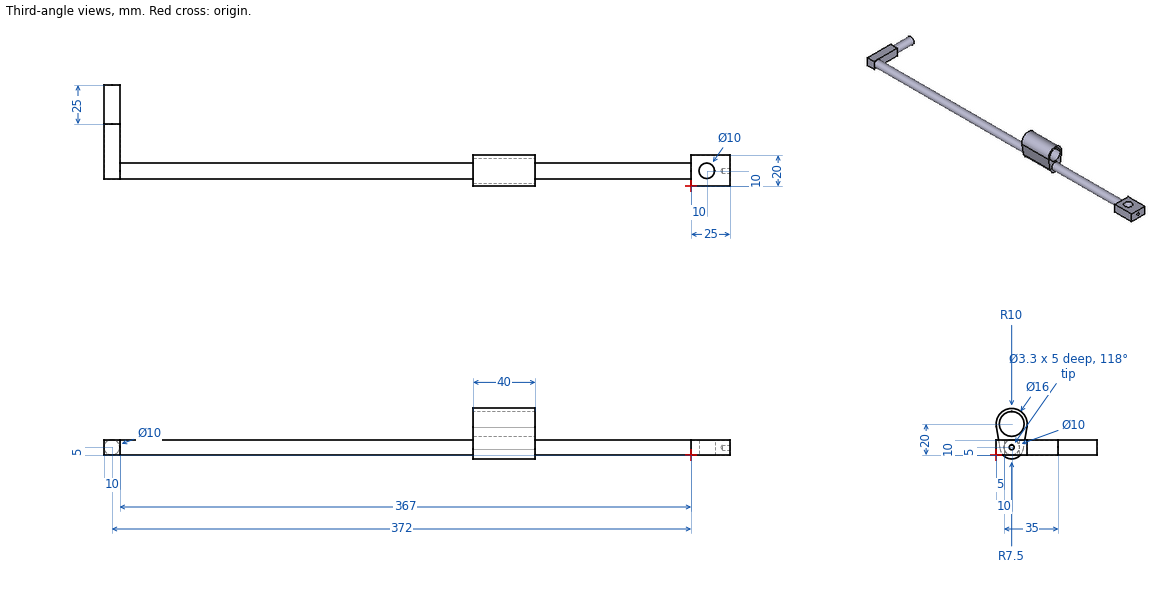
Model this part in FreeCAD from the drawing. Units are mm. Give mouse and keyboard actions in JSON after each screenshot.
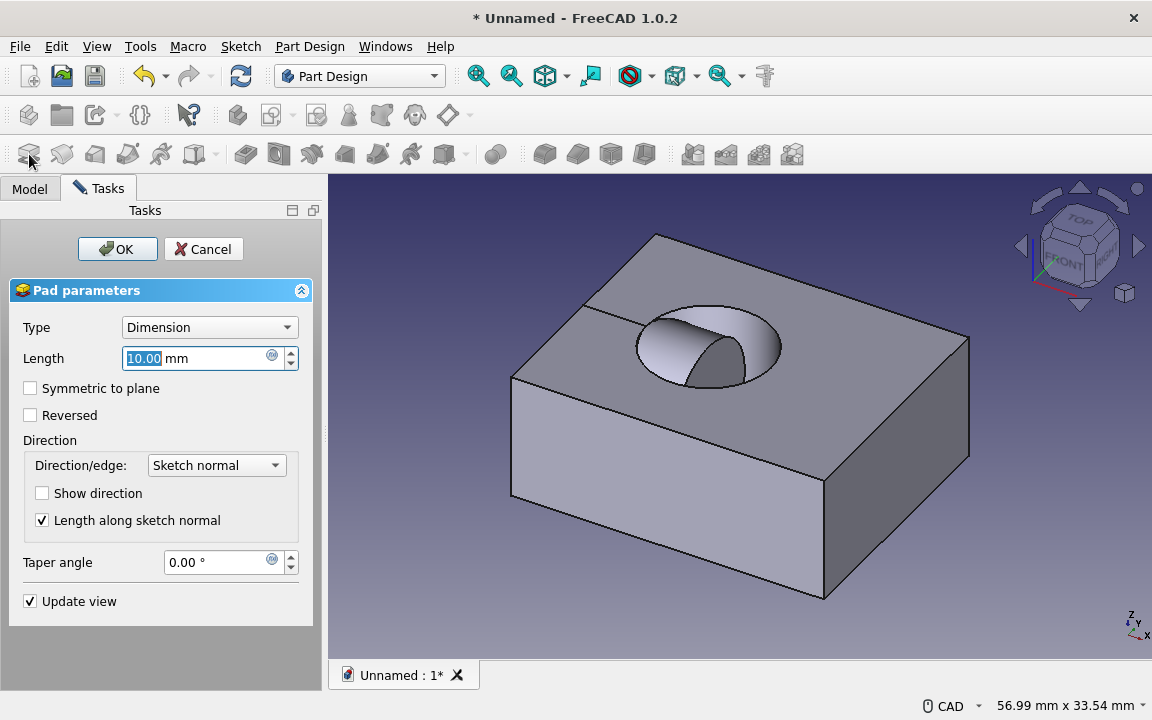
{"action": "type", "text": "367"}
{"action": "key", "text": "Tab"}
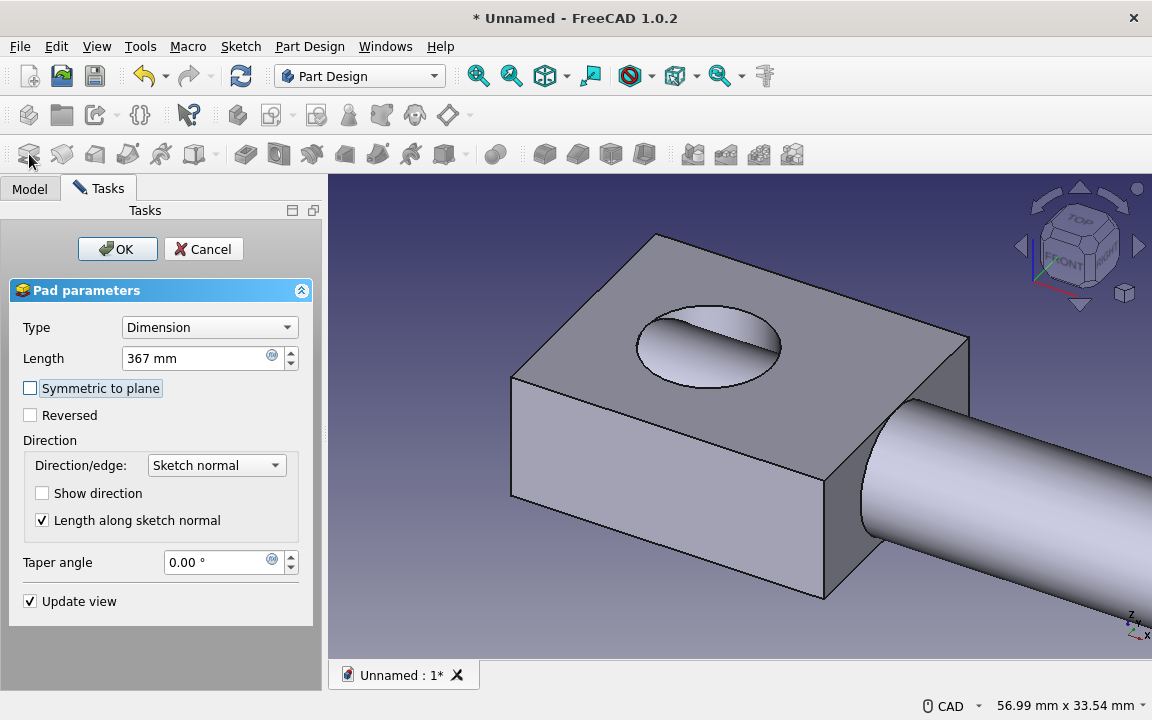
{"action": "left_click", "coordinate": [31, 415]}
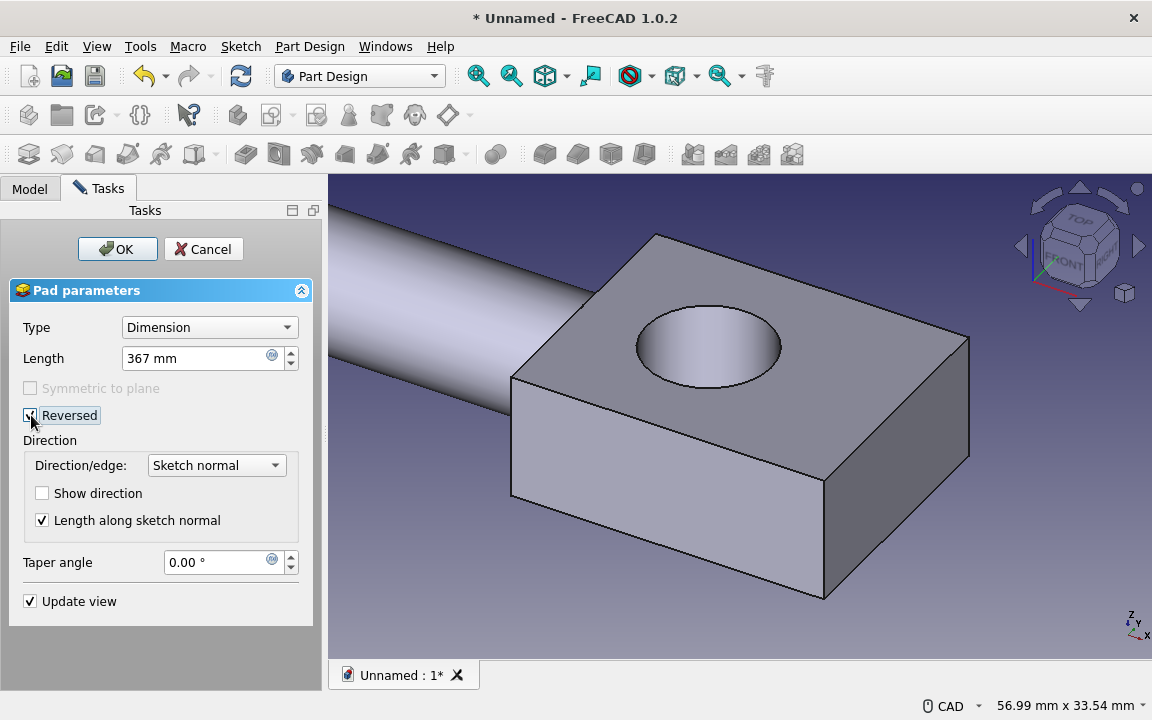
{"action": "left_click", "coordinate": [118, 249]}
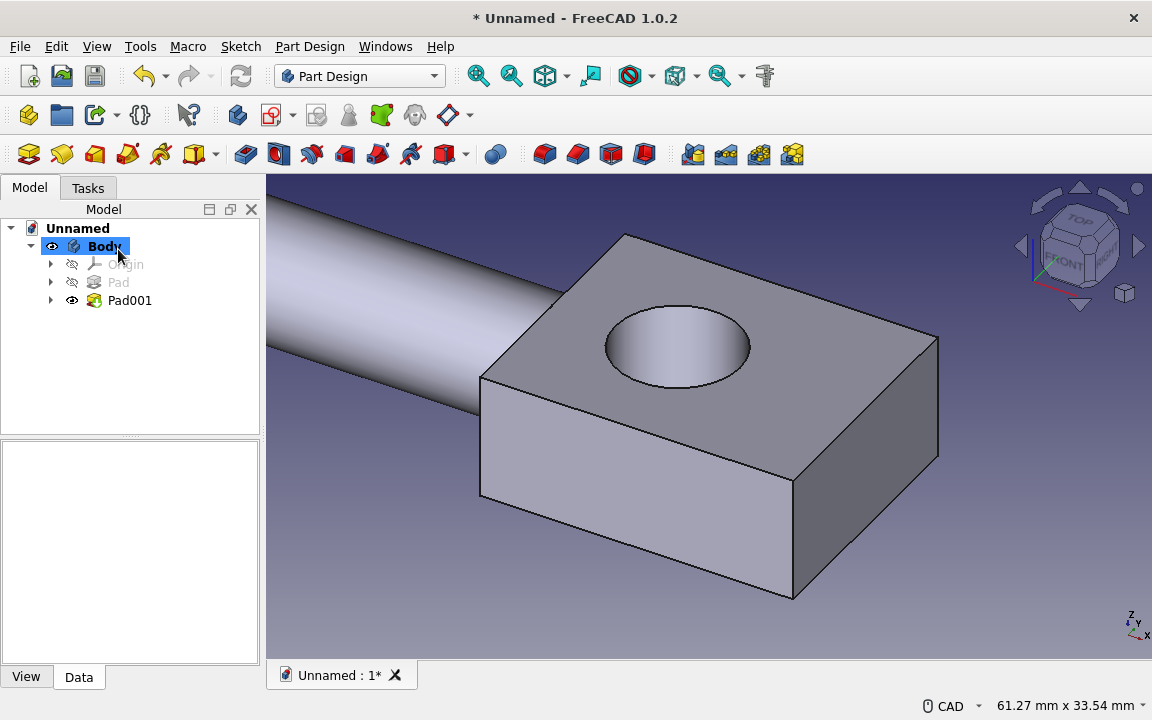
{"action": "key", "text": "v f"}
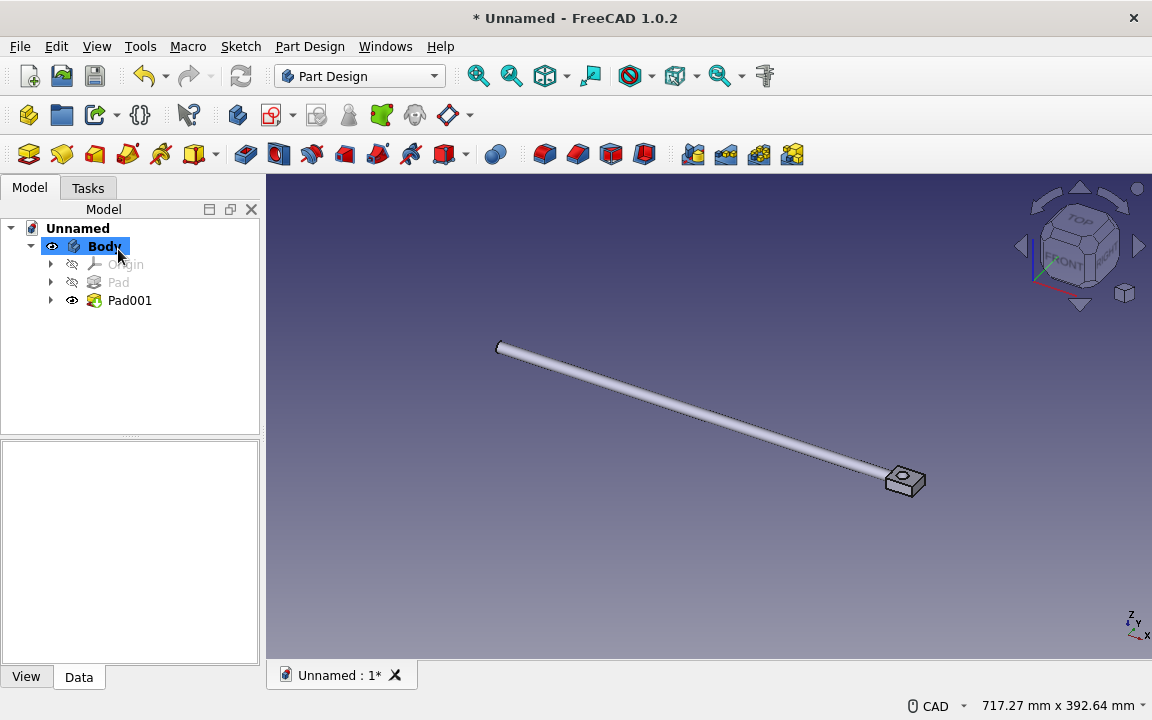
{"action": "scroll", "coordinate": [920, 483], "scroll_direction": "up", "scroll_amount": 4}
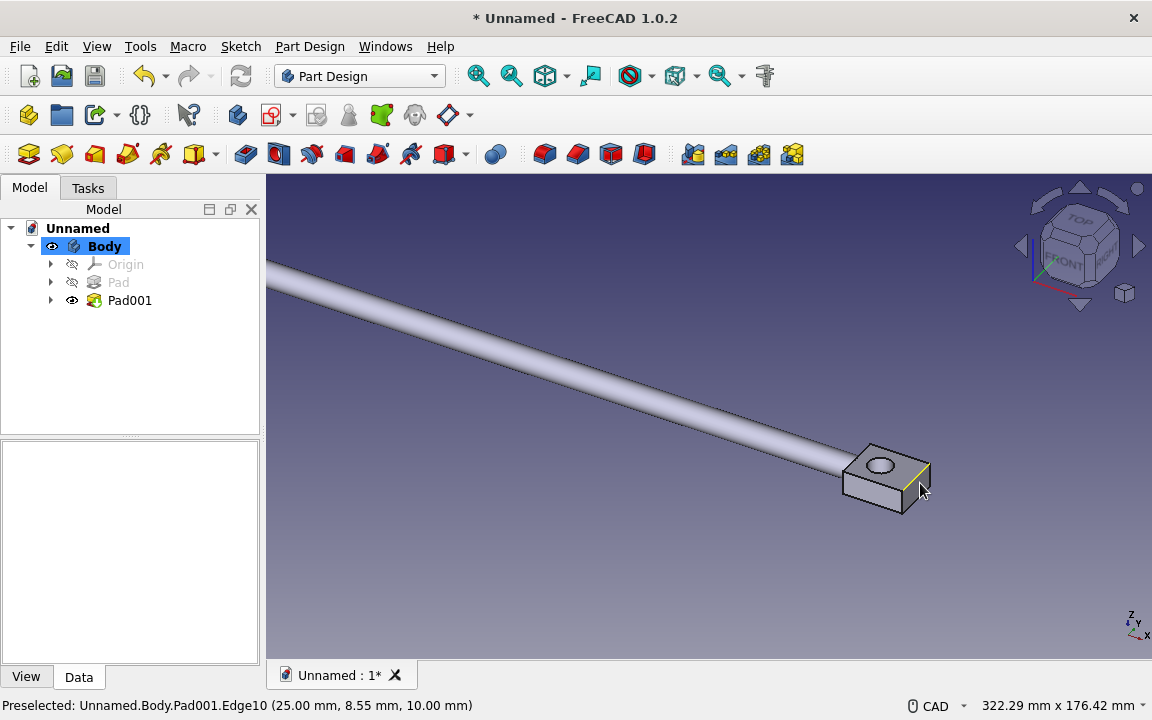
{"action": "left_click", "coordinate": [924, 483]}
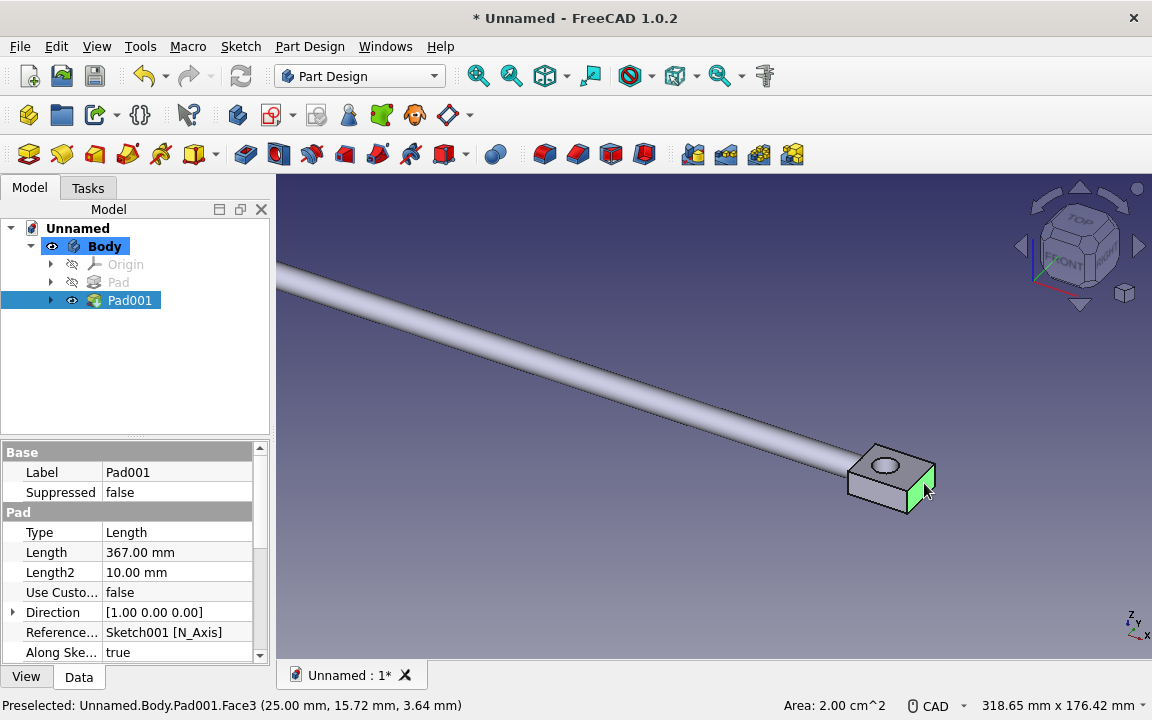
{"action": "left_click", "coordinate": [270, 116]}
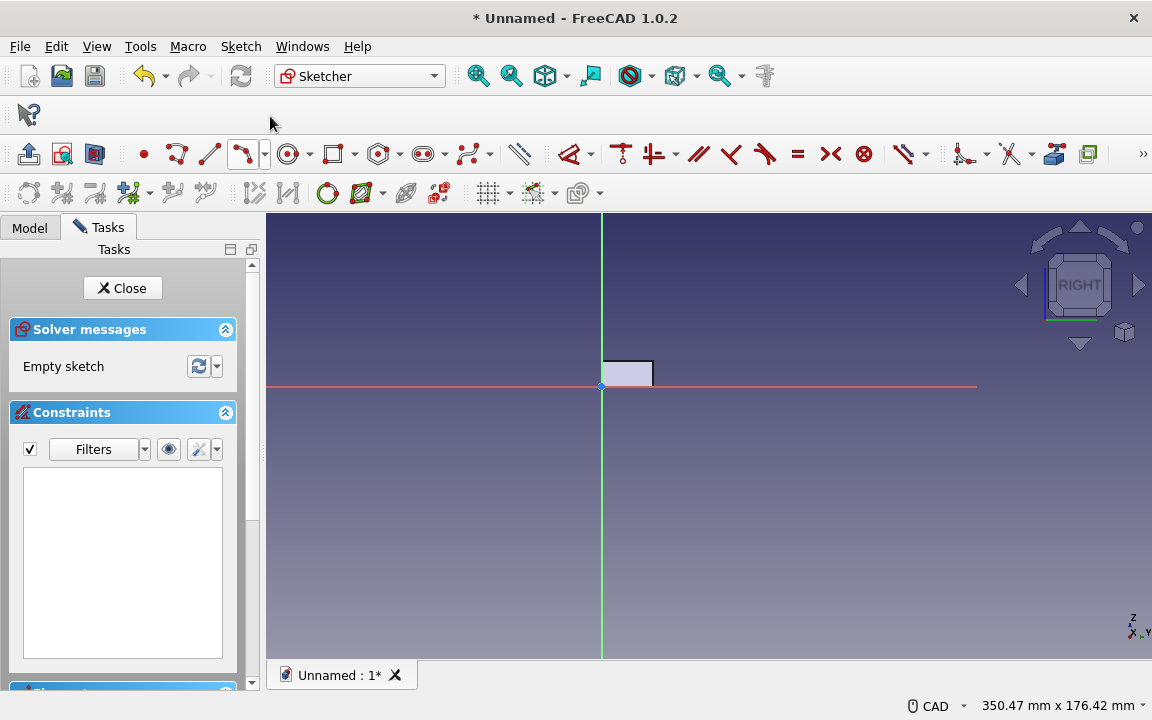
{"action": "scroll", "coordinate": [627, 371], "scroll_direction": "up", "scroll_amount": 15}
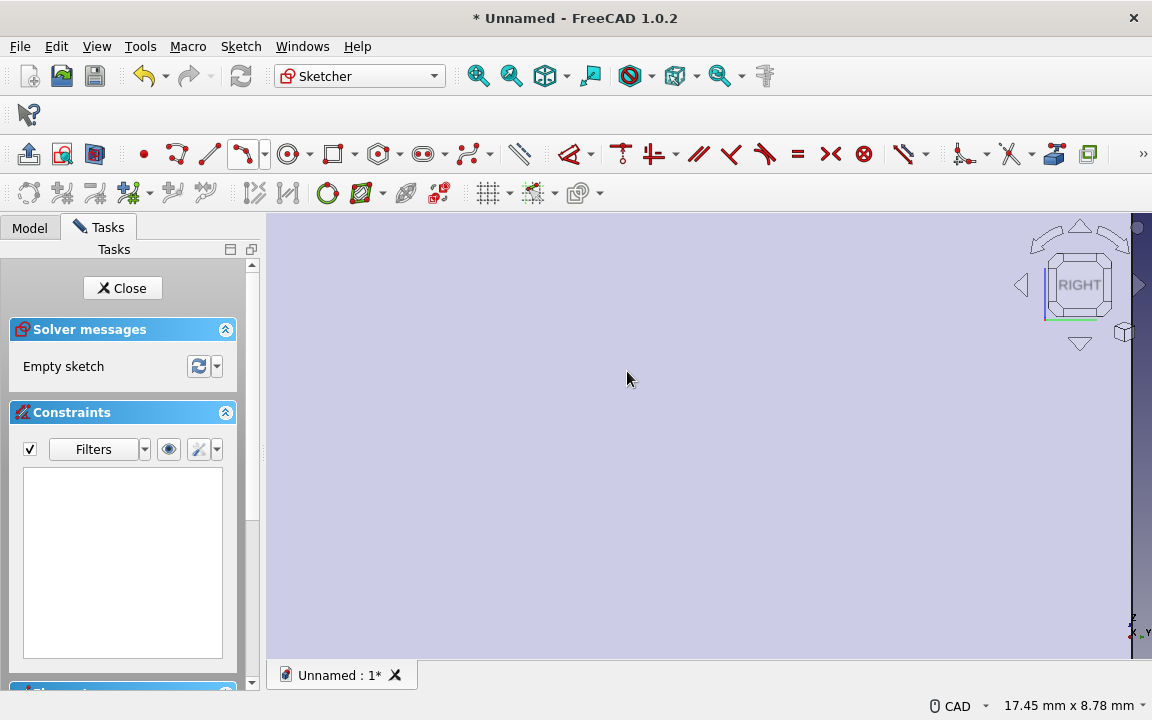
{"action": "scroll", "coordinate": [592, 402], "scroll_direction": "up", "scroll_amount": 2}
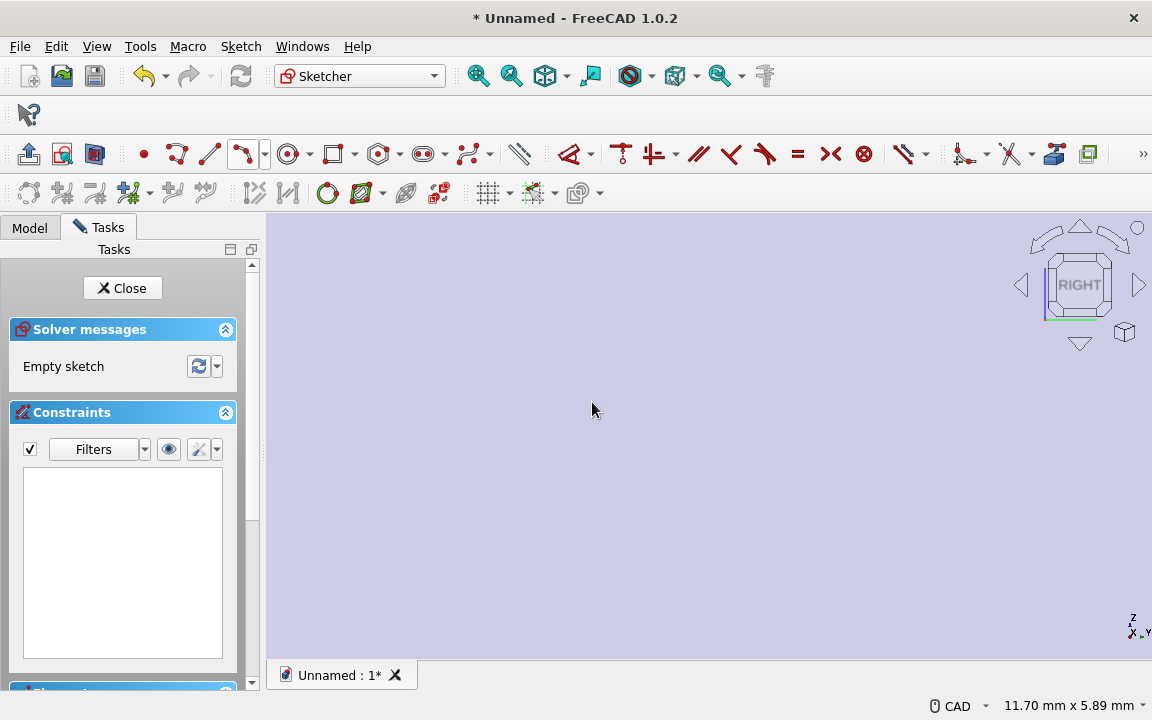
{"action": "left_click", "coordinate": [288, 154]}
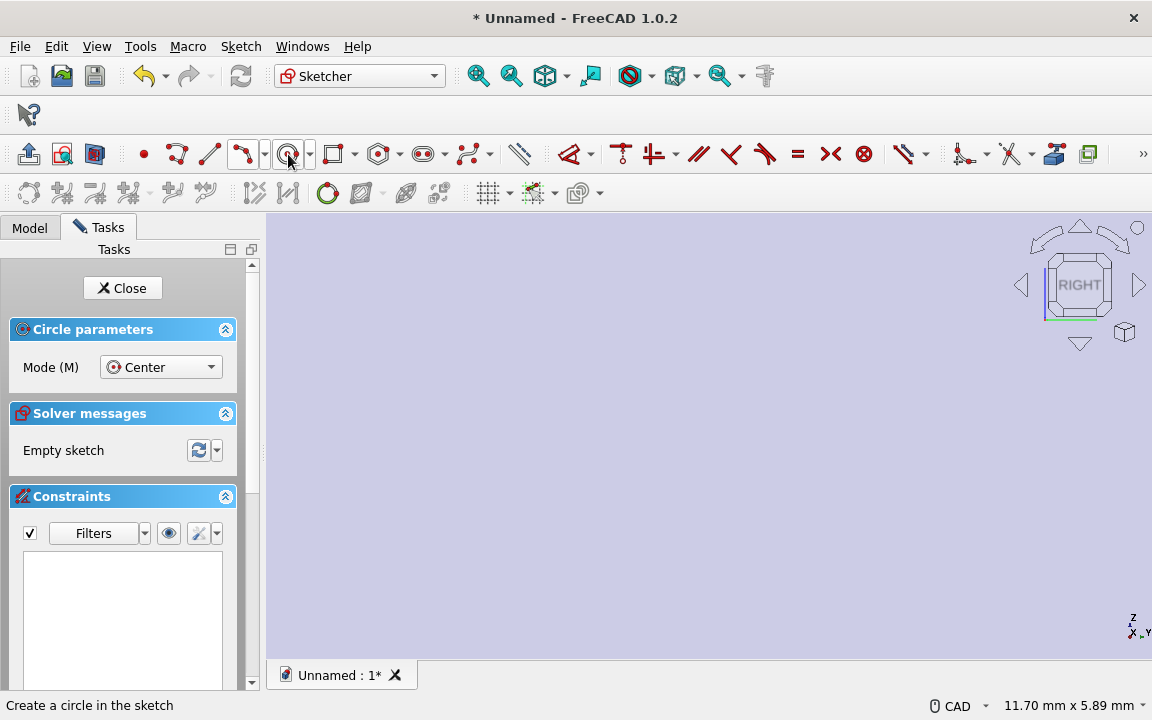
{"action": "left_click", "coordinate": [641, 436]}
{"action": "mouse_move", "coordinate": [729, 348]}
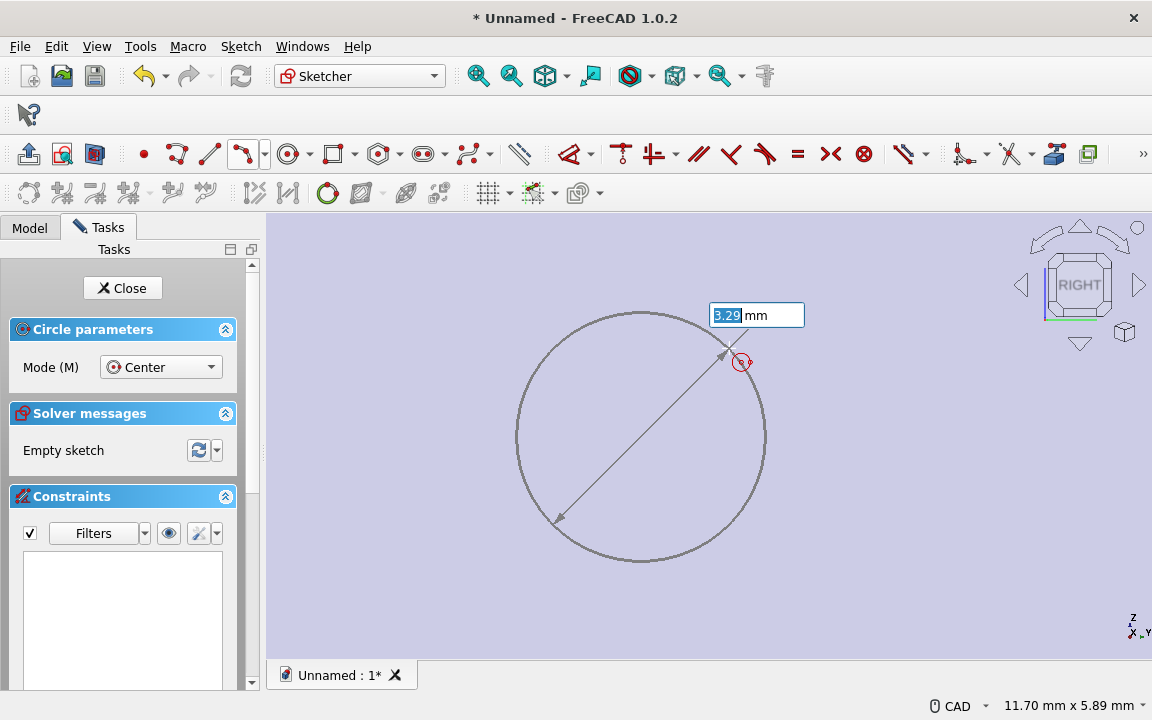
{"action": "type", "text": "3.3"}
{"action": "key", "text": "Return"}
{"action": "key", "text": "Escape"}